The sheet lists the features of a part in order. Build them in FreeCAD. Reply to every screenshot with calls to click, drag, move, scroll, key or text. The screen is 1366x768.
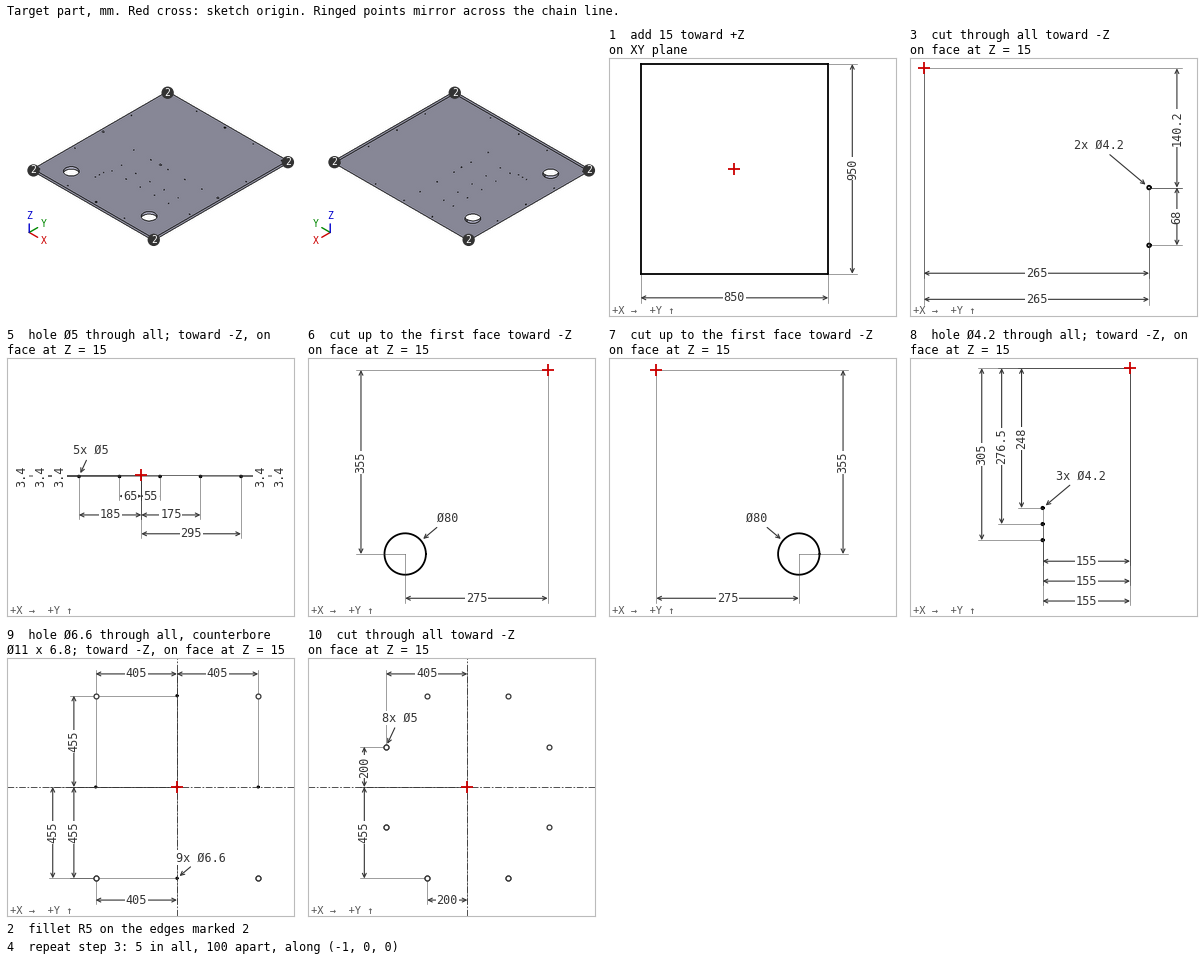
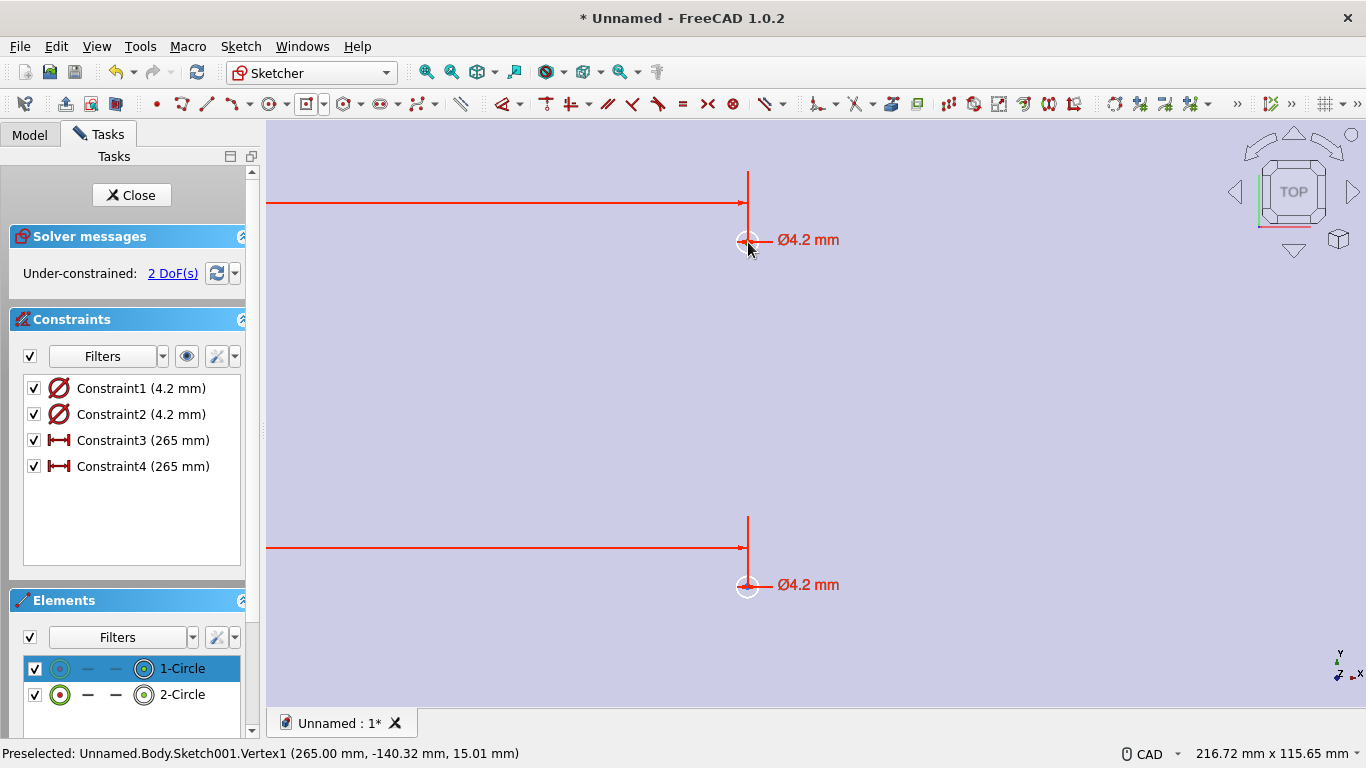
click(748, 587)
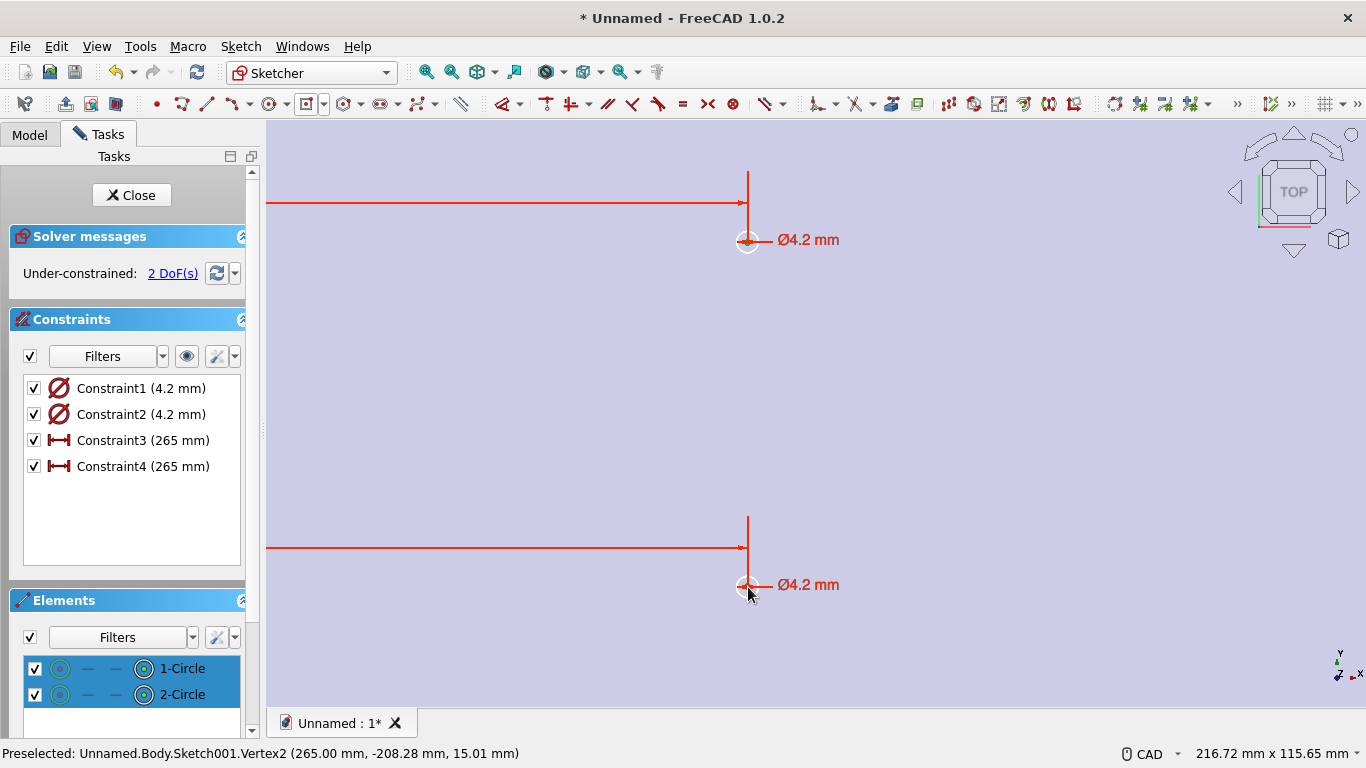
click(520, 104)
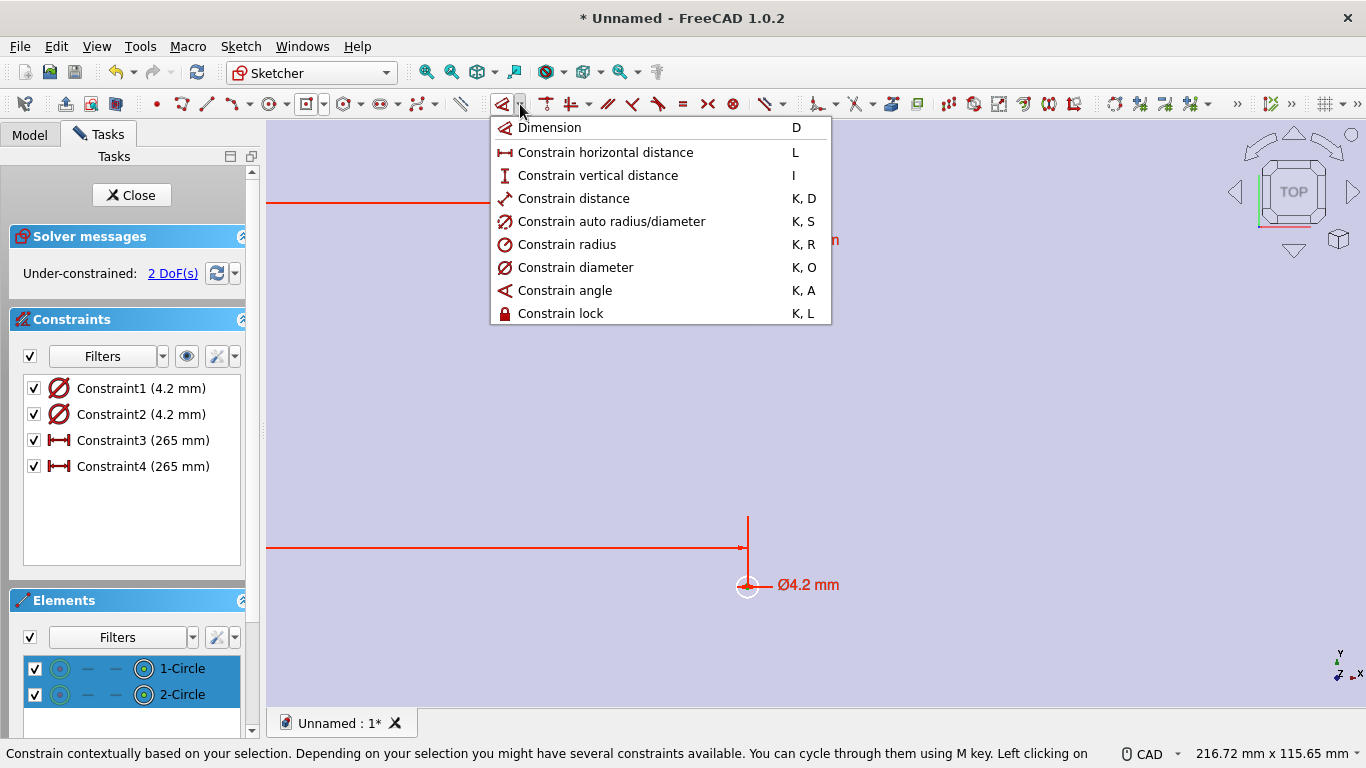
click(661, 176)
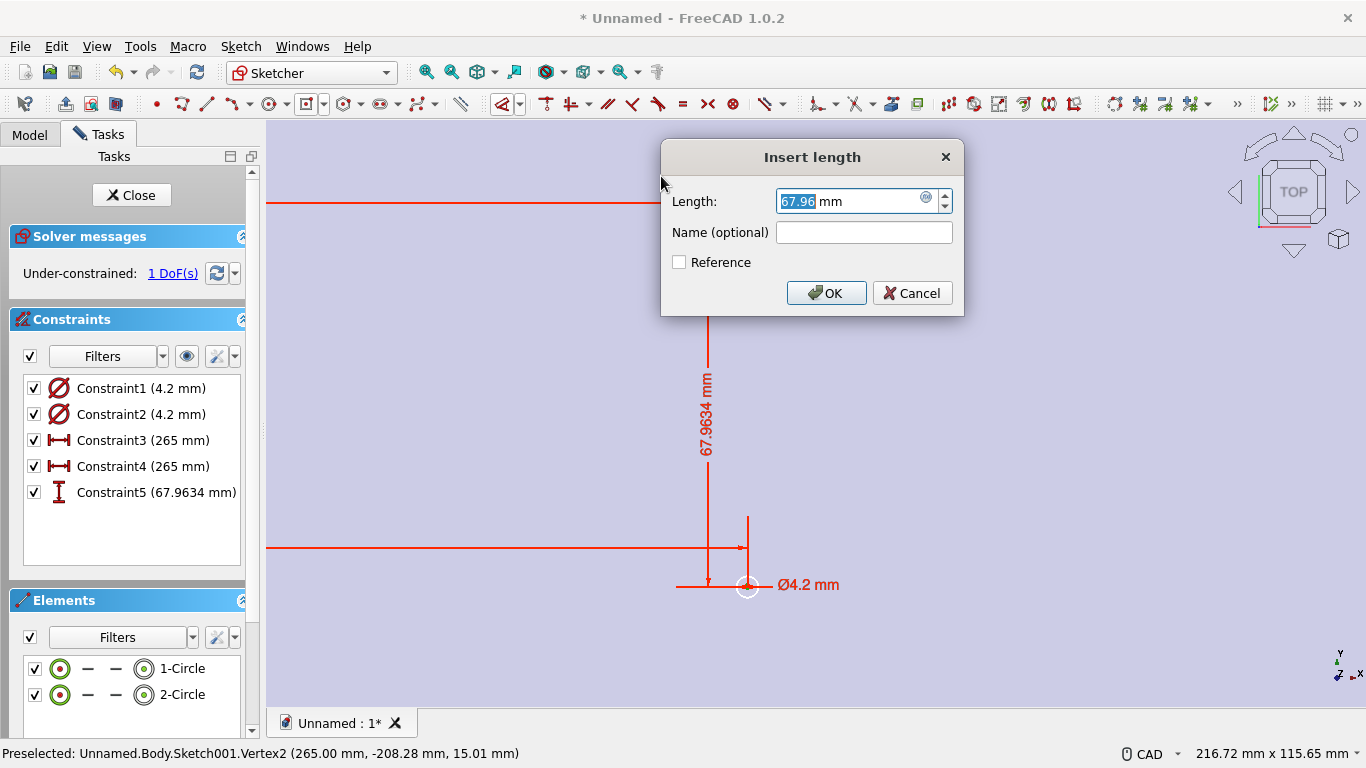
text(68)
key(Return)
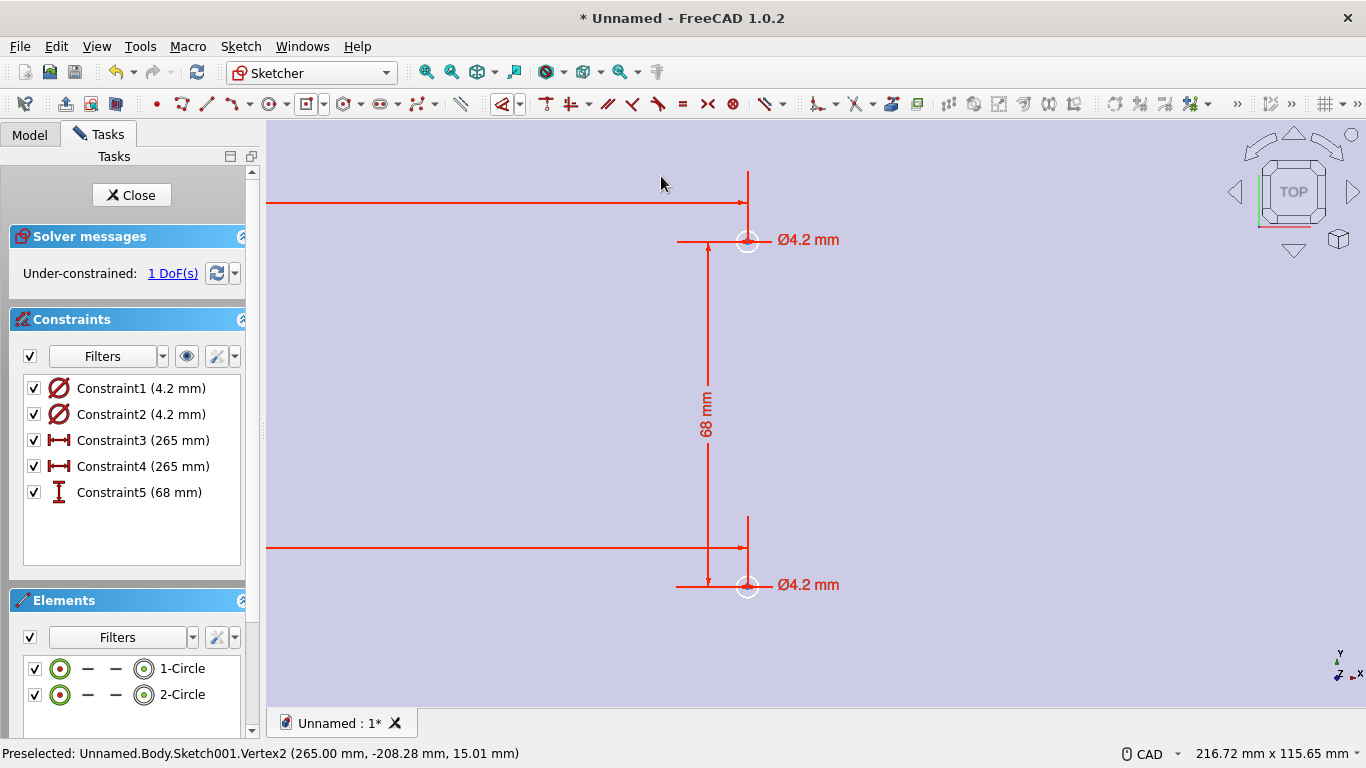
click(748, 242)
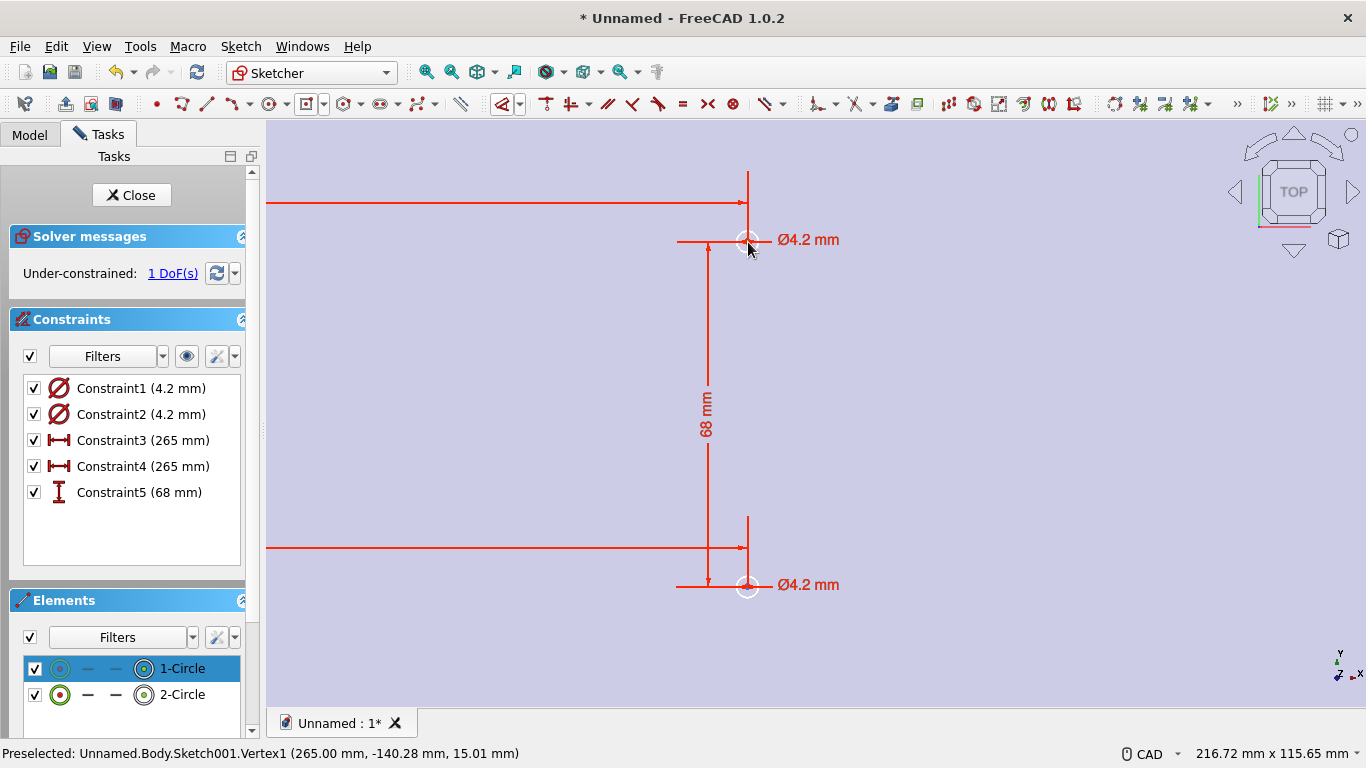
click(520, 104)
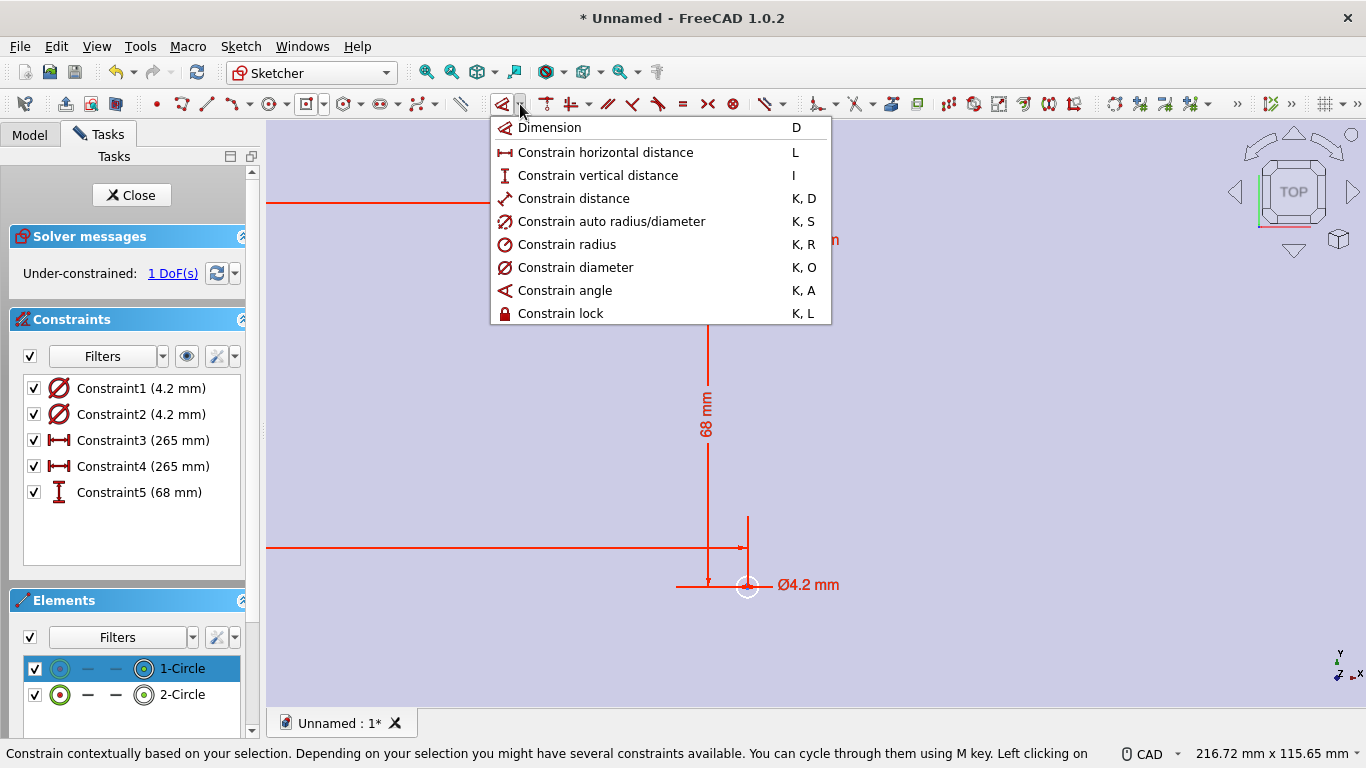
click(661, 176)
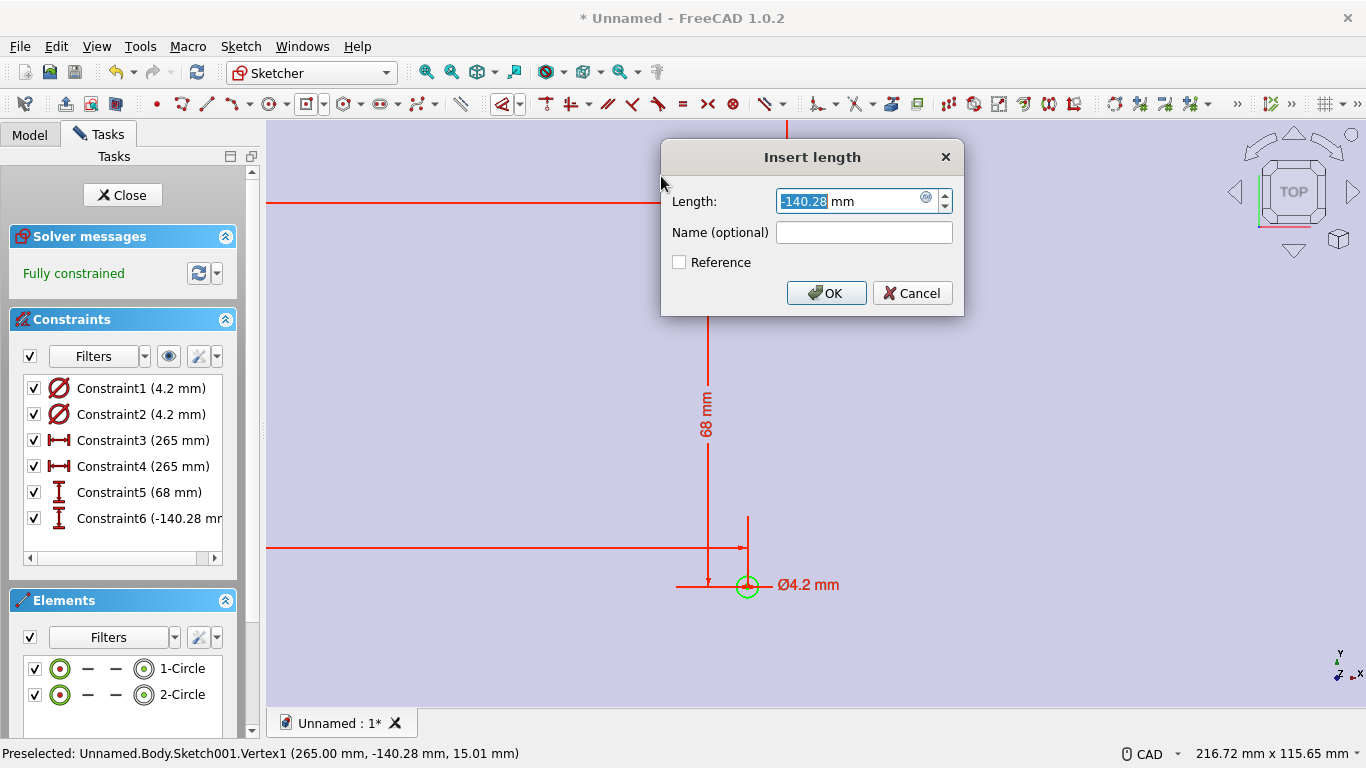
text(-140.2)
key(Return)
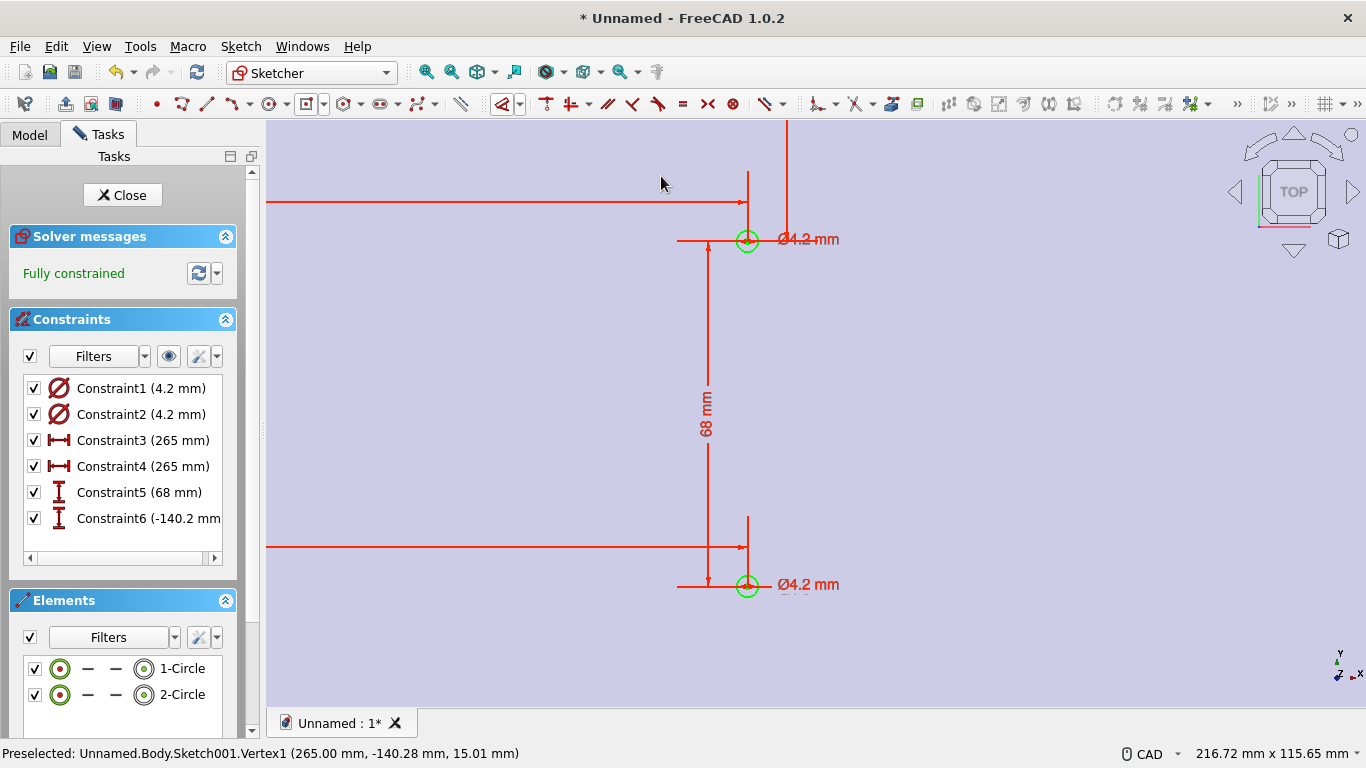
click(123, 195)